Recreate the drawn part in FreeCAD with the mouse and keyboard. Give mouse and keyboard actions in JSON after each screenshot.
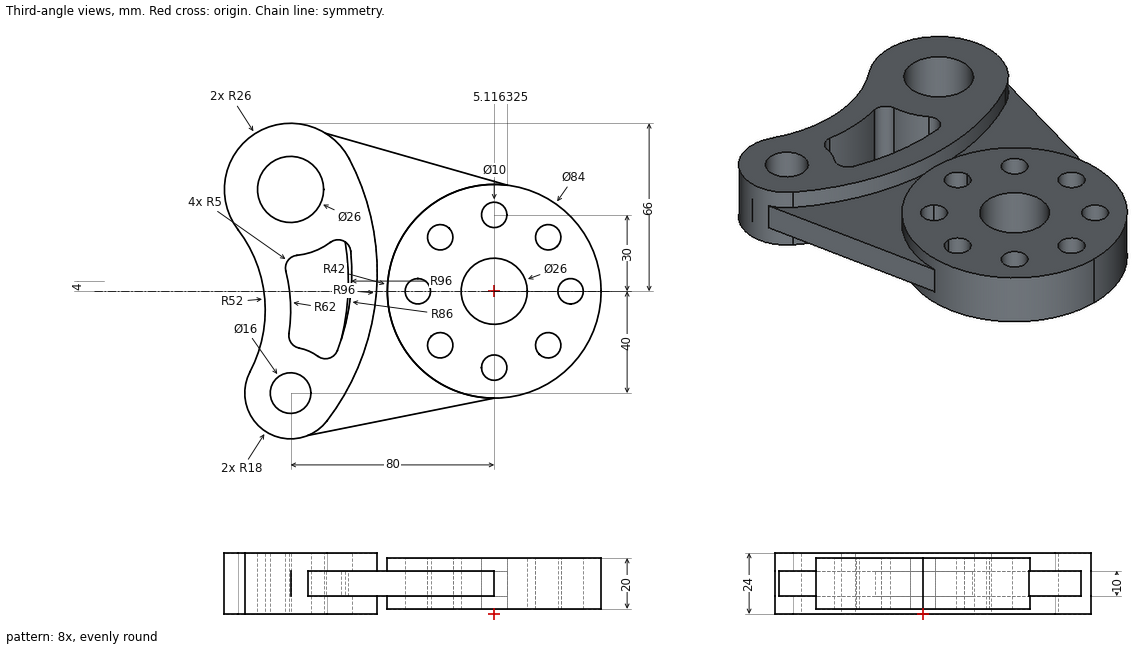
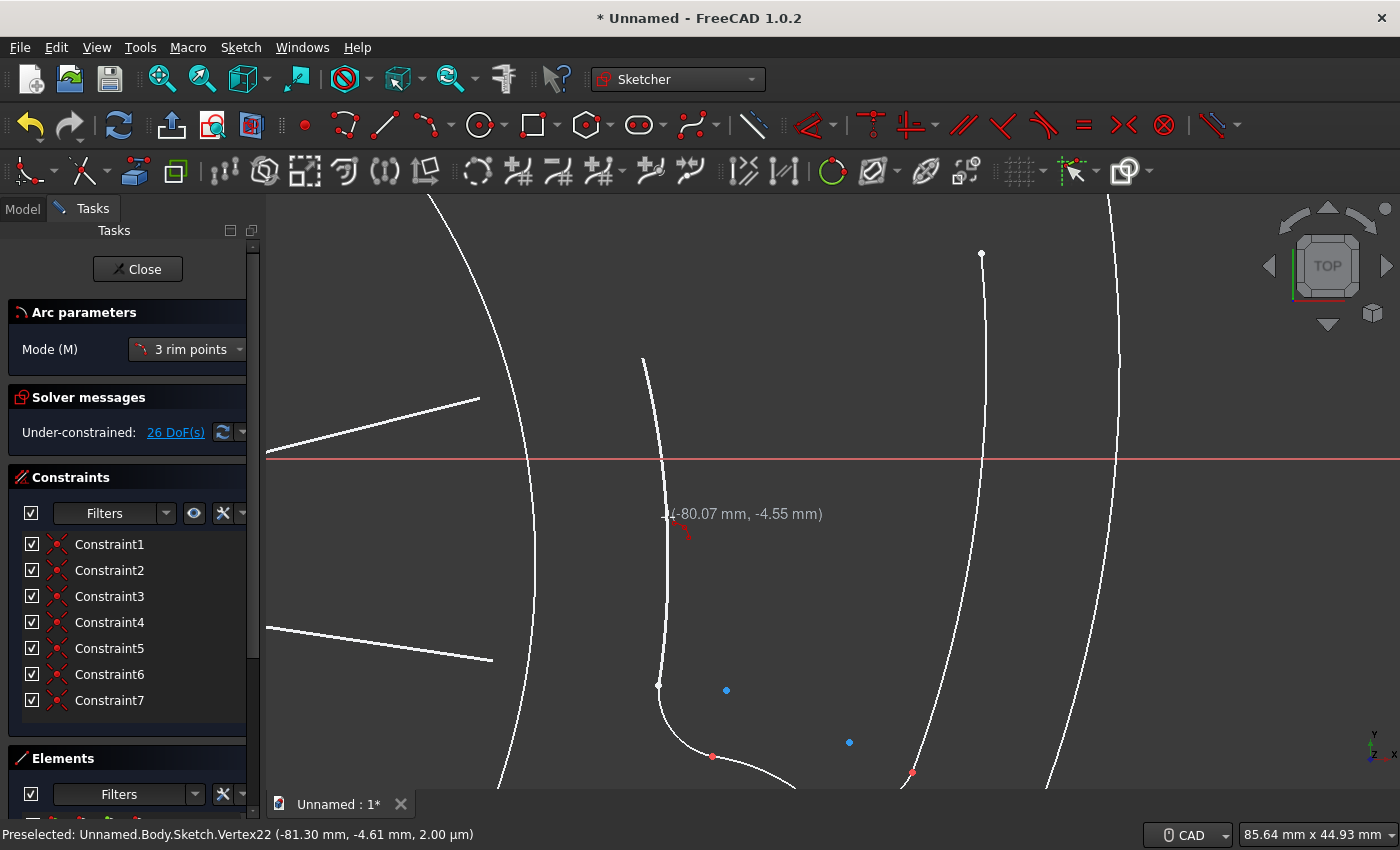
{"action": "left_click", "coordinate": [668, 516]}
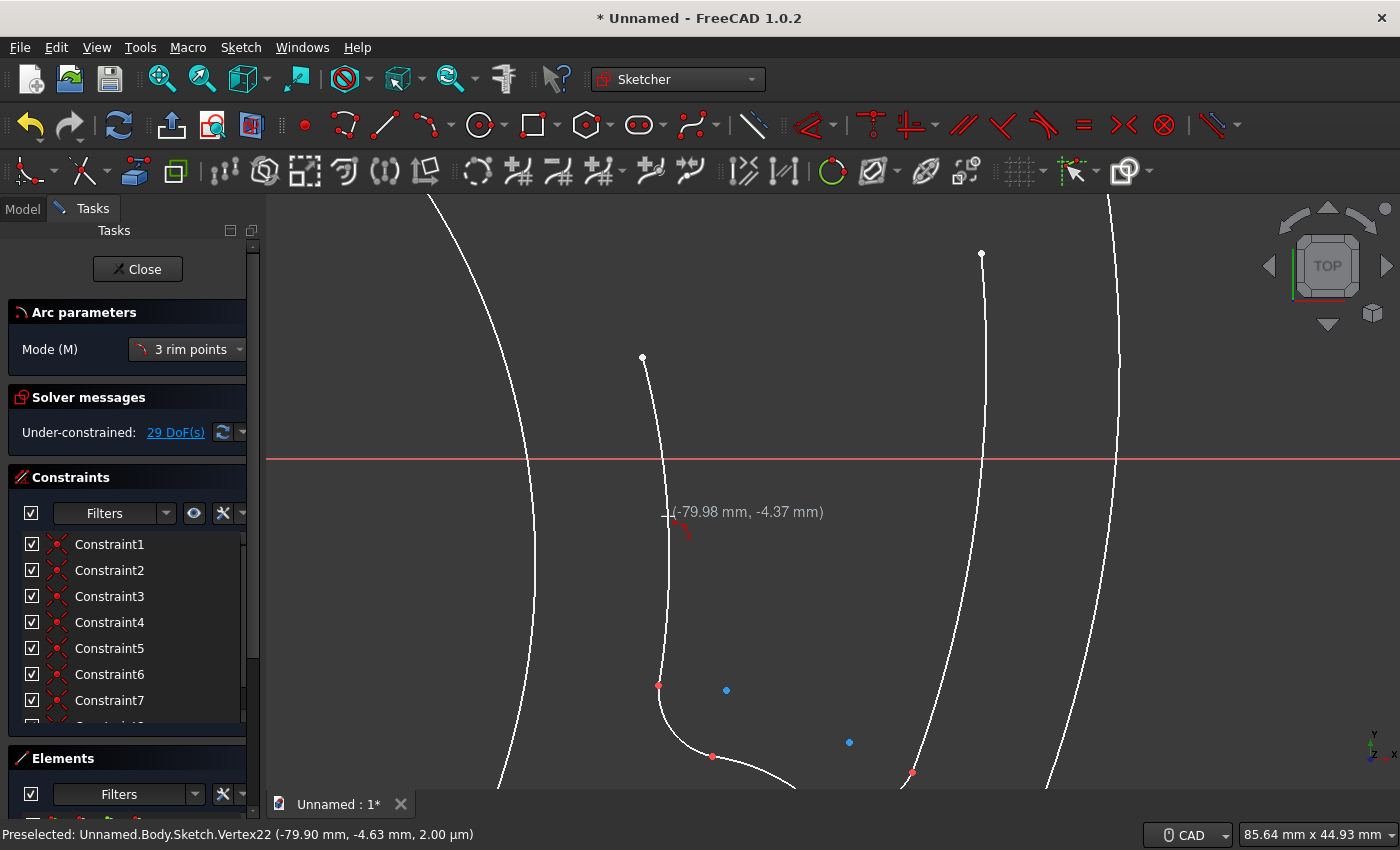
{"action": "scroll", "coordinate": [668, 517], "scroll_direction": "down", "scroll_amount": 7}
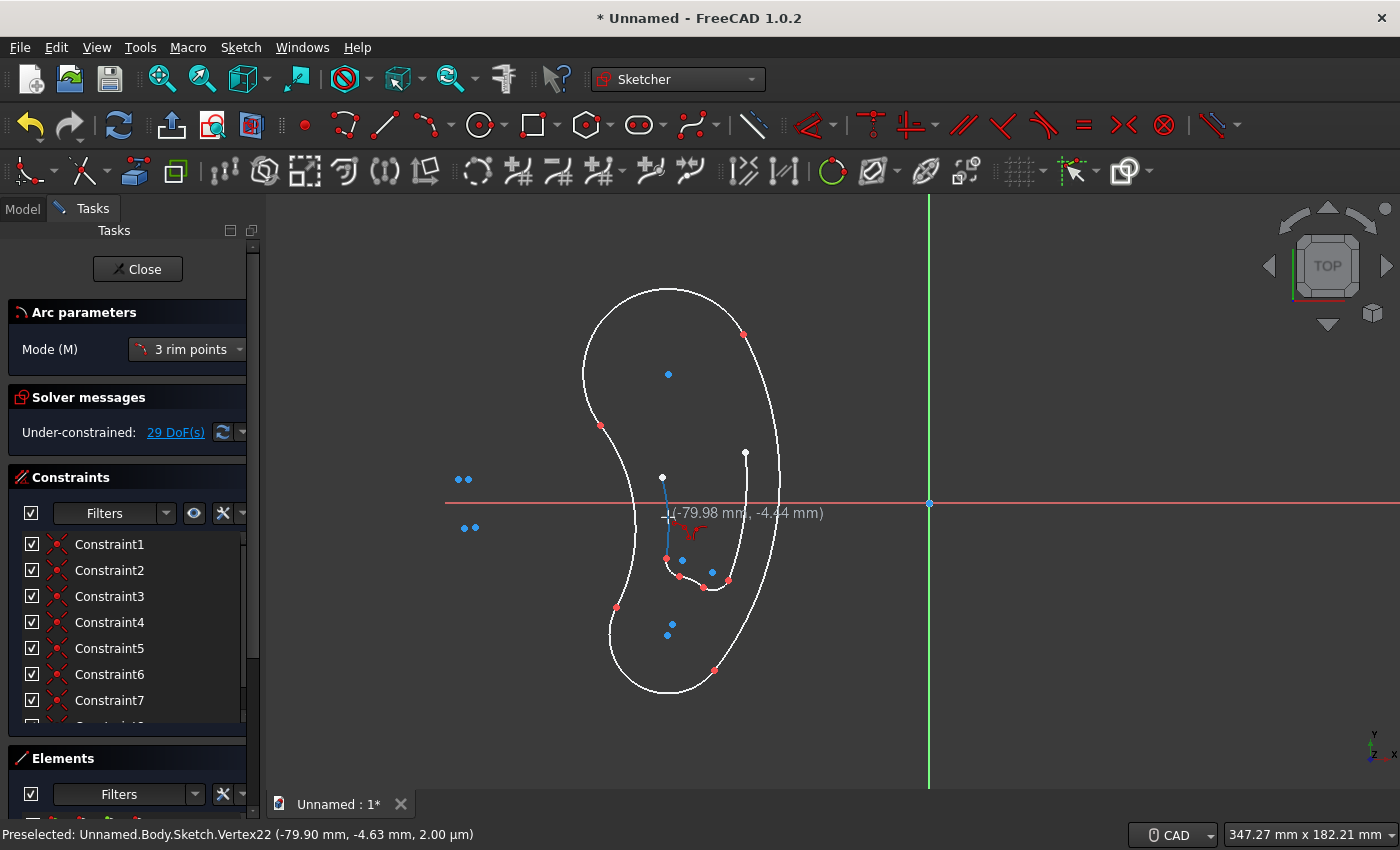
{"action": "left_click", "coordinate": [662, 478]}
{"action": "left_click", "coordinate": [676, 457]}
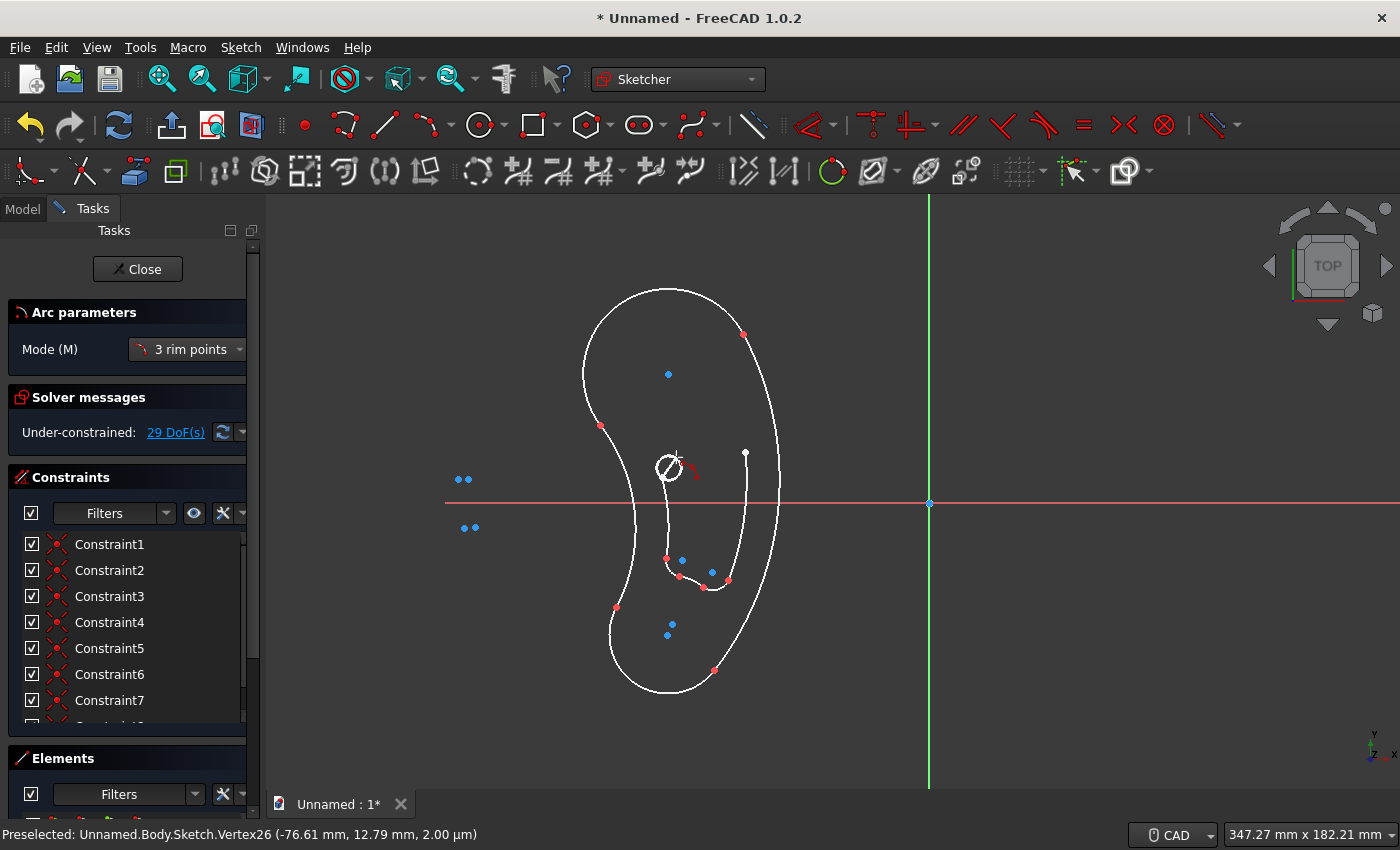
{"action": "scroll", "coordinate": [665, 464], "scroll_direction": "up", "scroll_amount": 6}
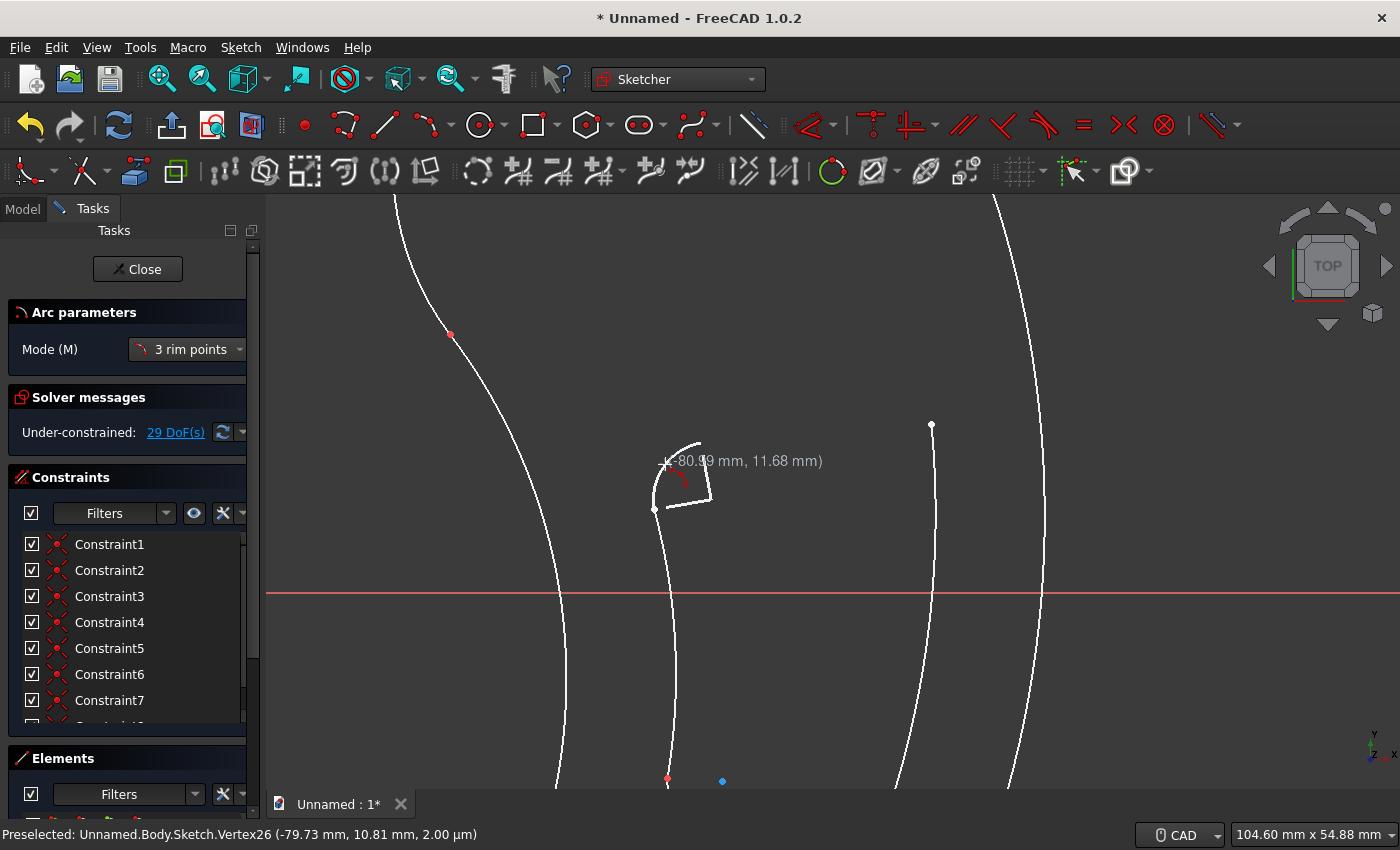
{"action": "left_click", "coordinate": [663, 463]}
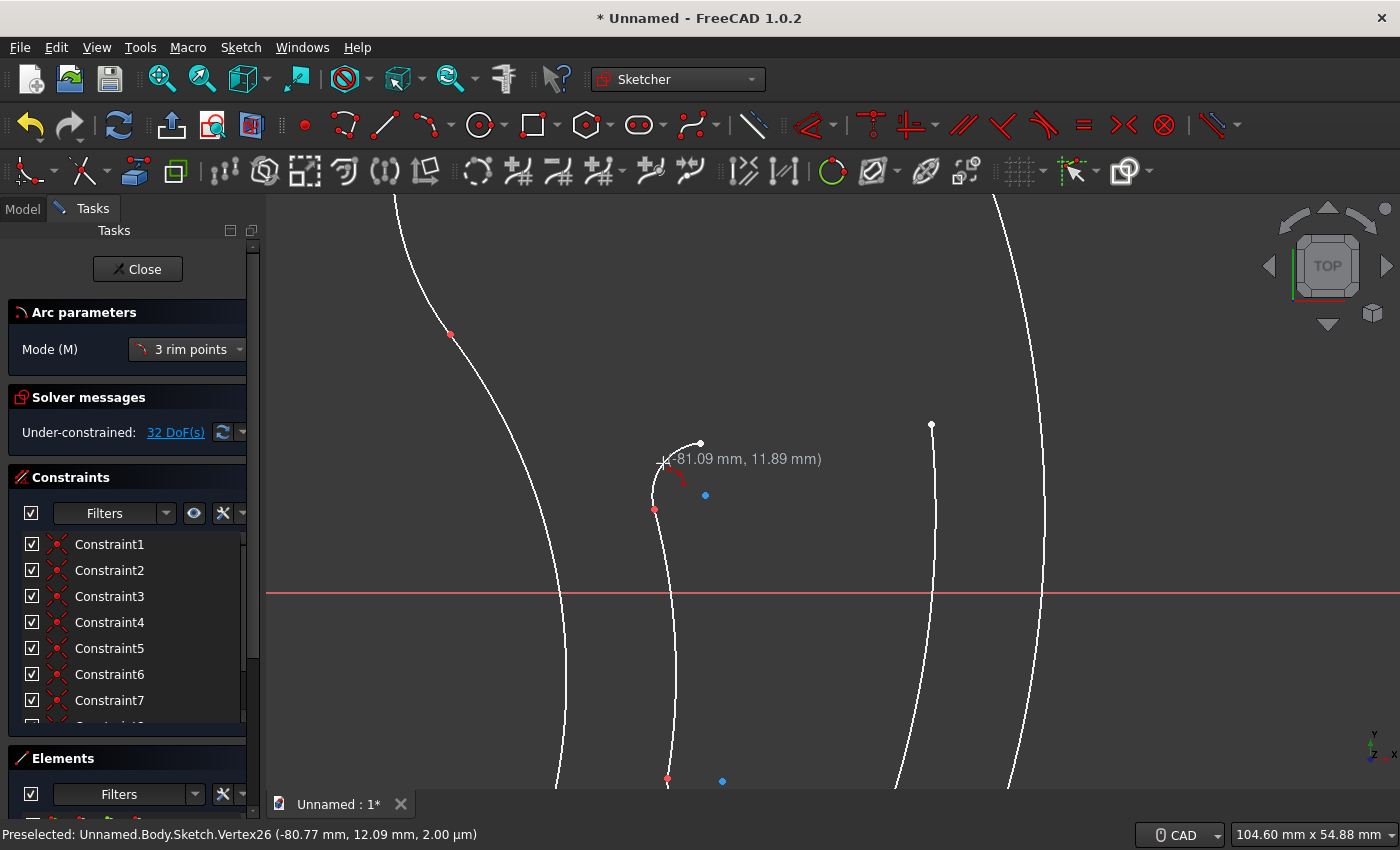
{"action": "left_click", "coordinate": [701, 443]}
{"action": "left_click", "coordinate": [845, 384]}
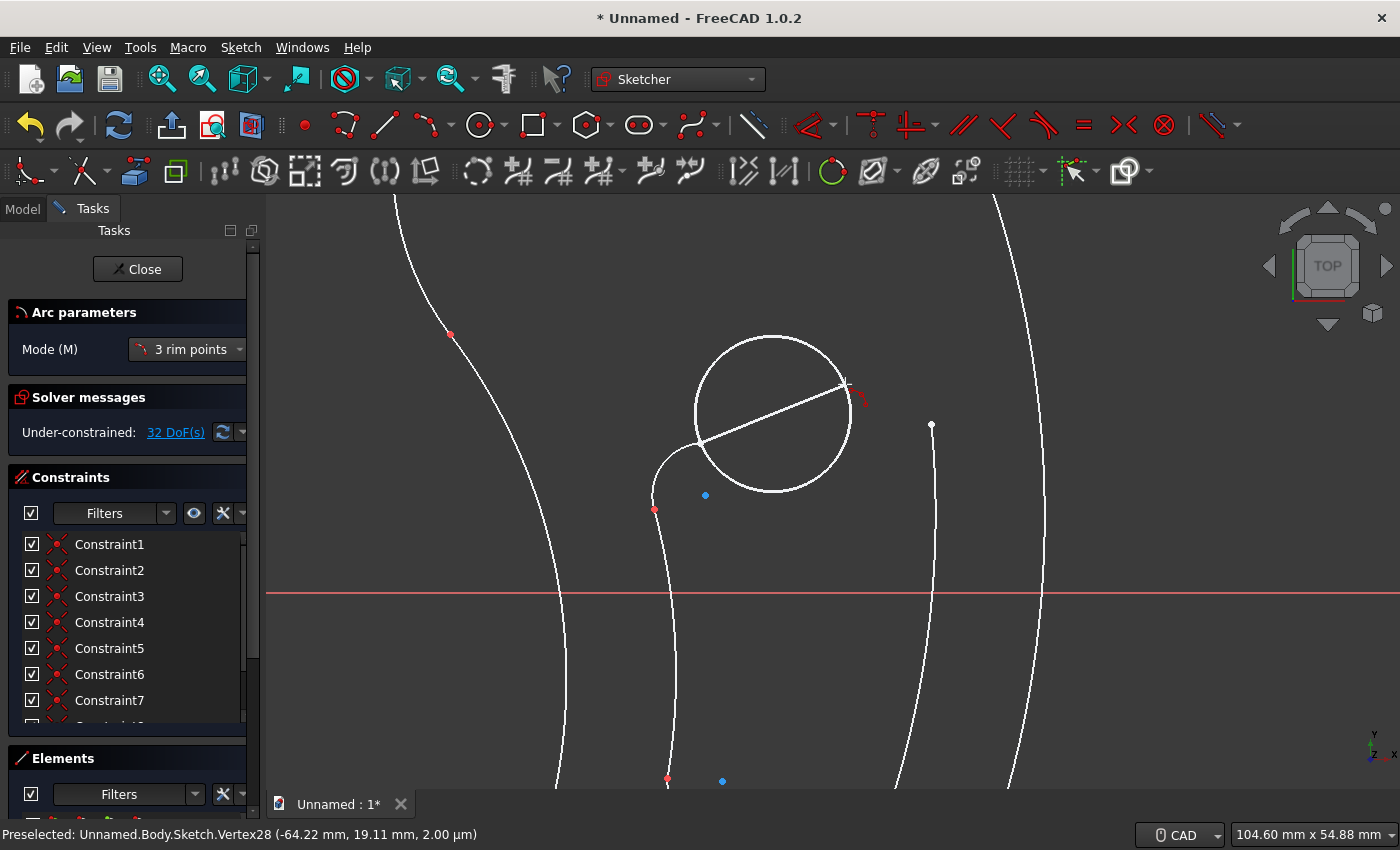
{"action": "scroll", "coordinate": [777, 422], "scroll_direction": "up", "scroll_amount": 3}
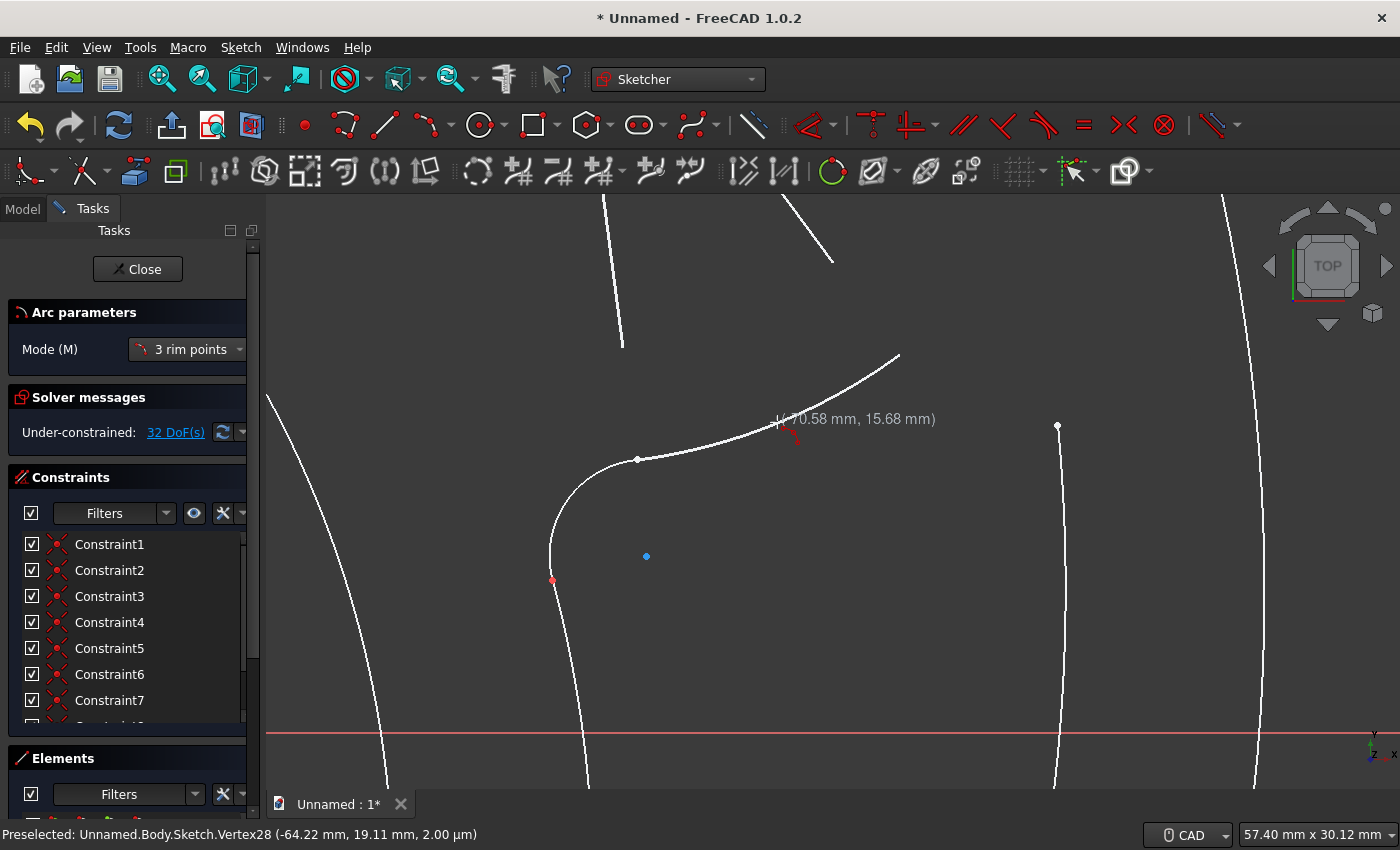
{"action": "left_click", "coordinate": [777, 422]}